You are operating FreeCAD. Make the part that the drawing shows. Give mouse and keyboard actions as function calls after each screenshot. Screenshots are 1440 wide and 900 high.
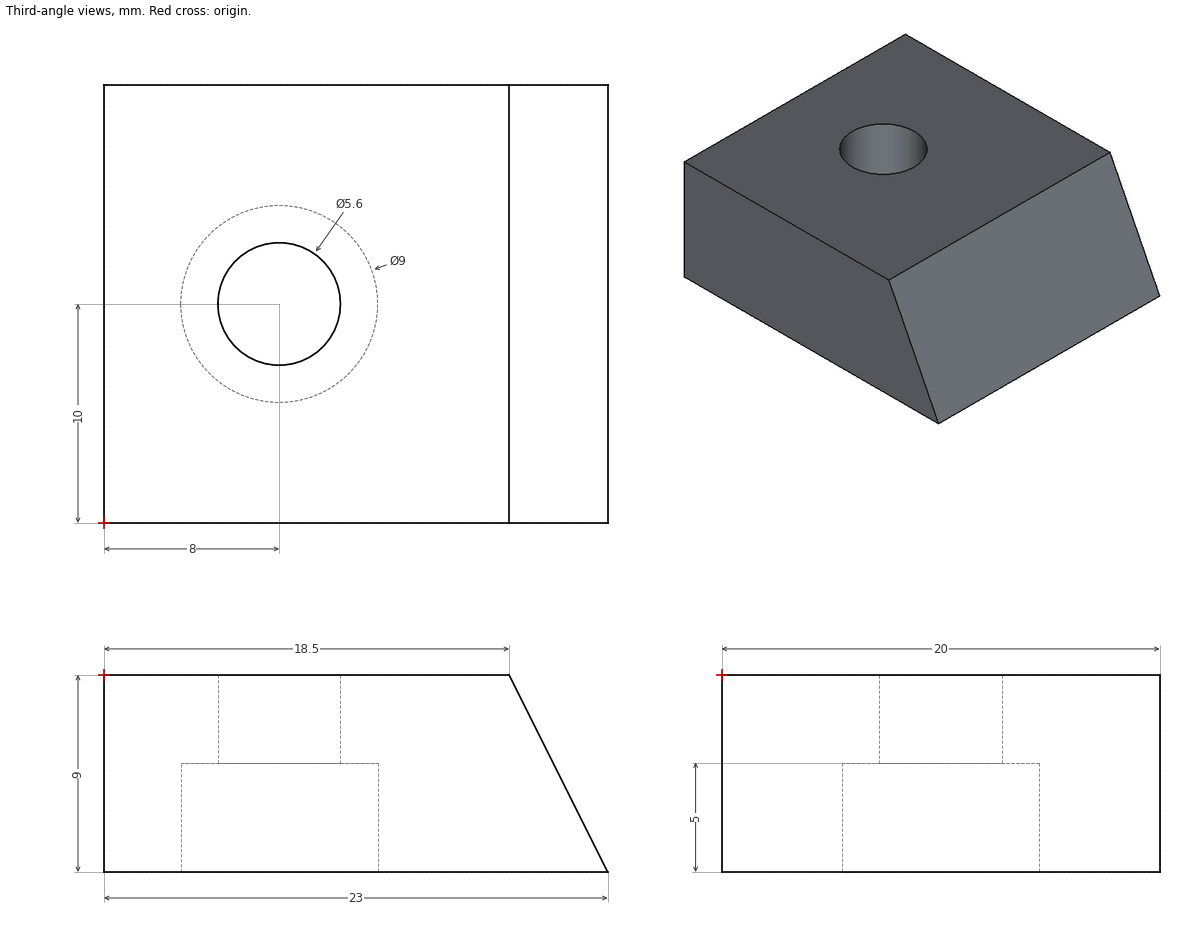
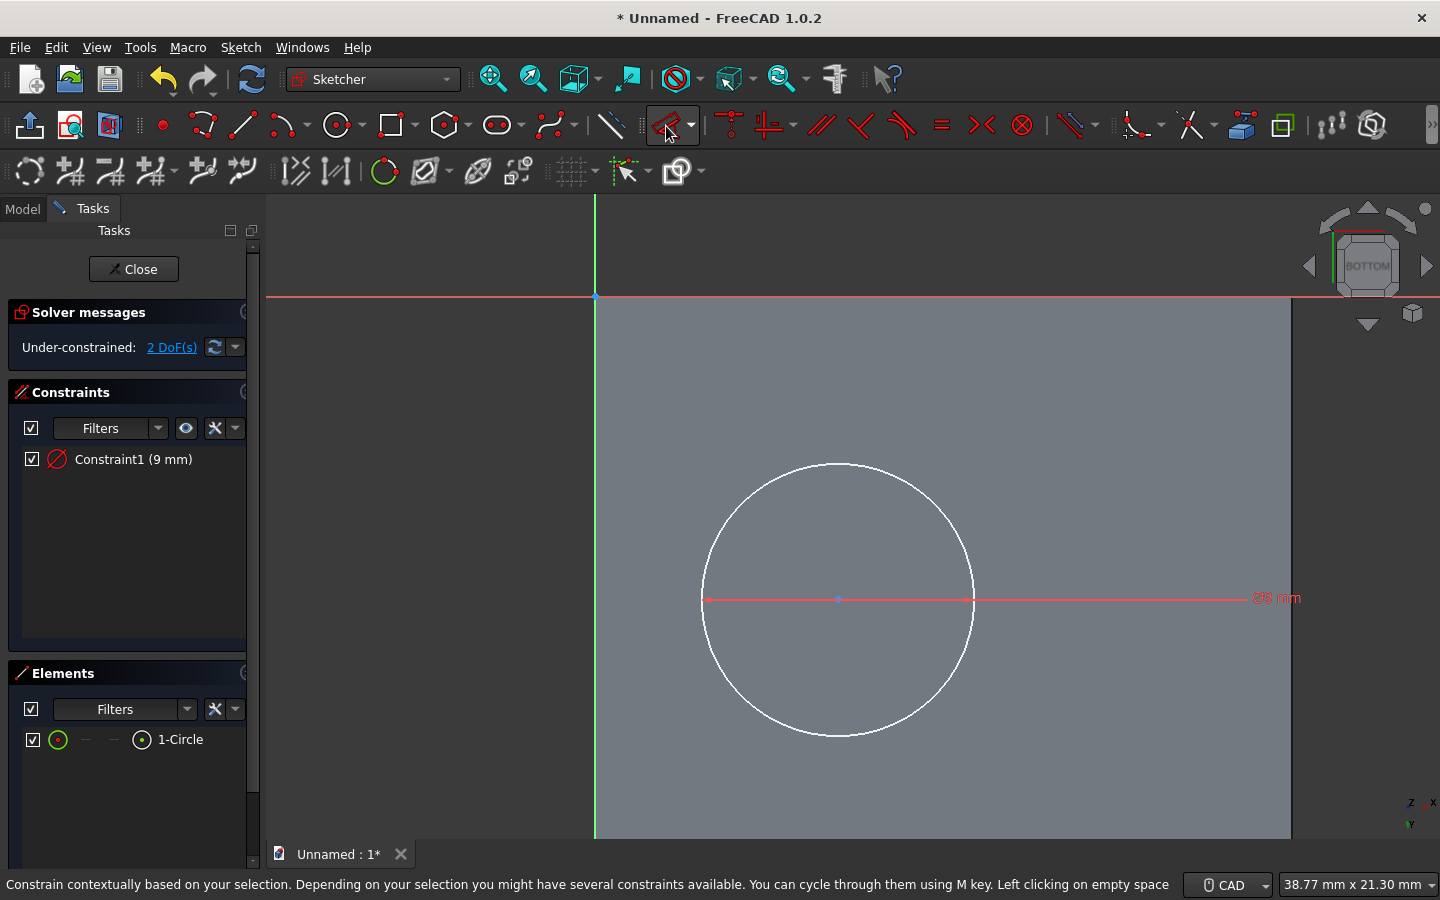
click(838, 600)
click(717, 263)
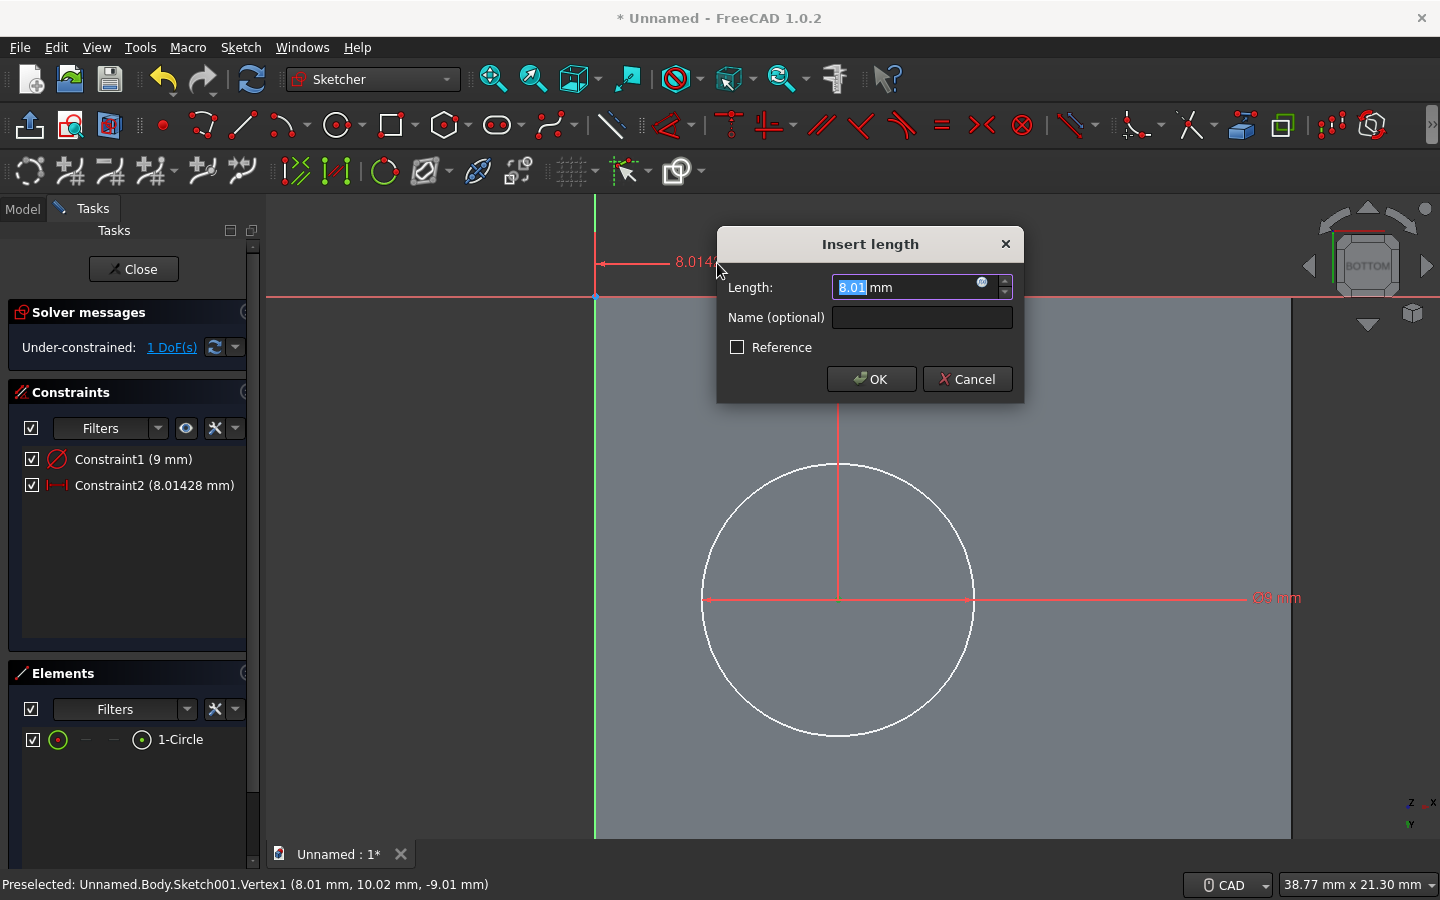
text(8)
key(Return)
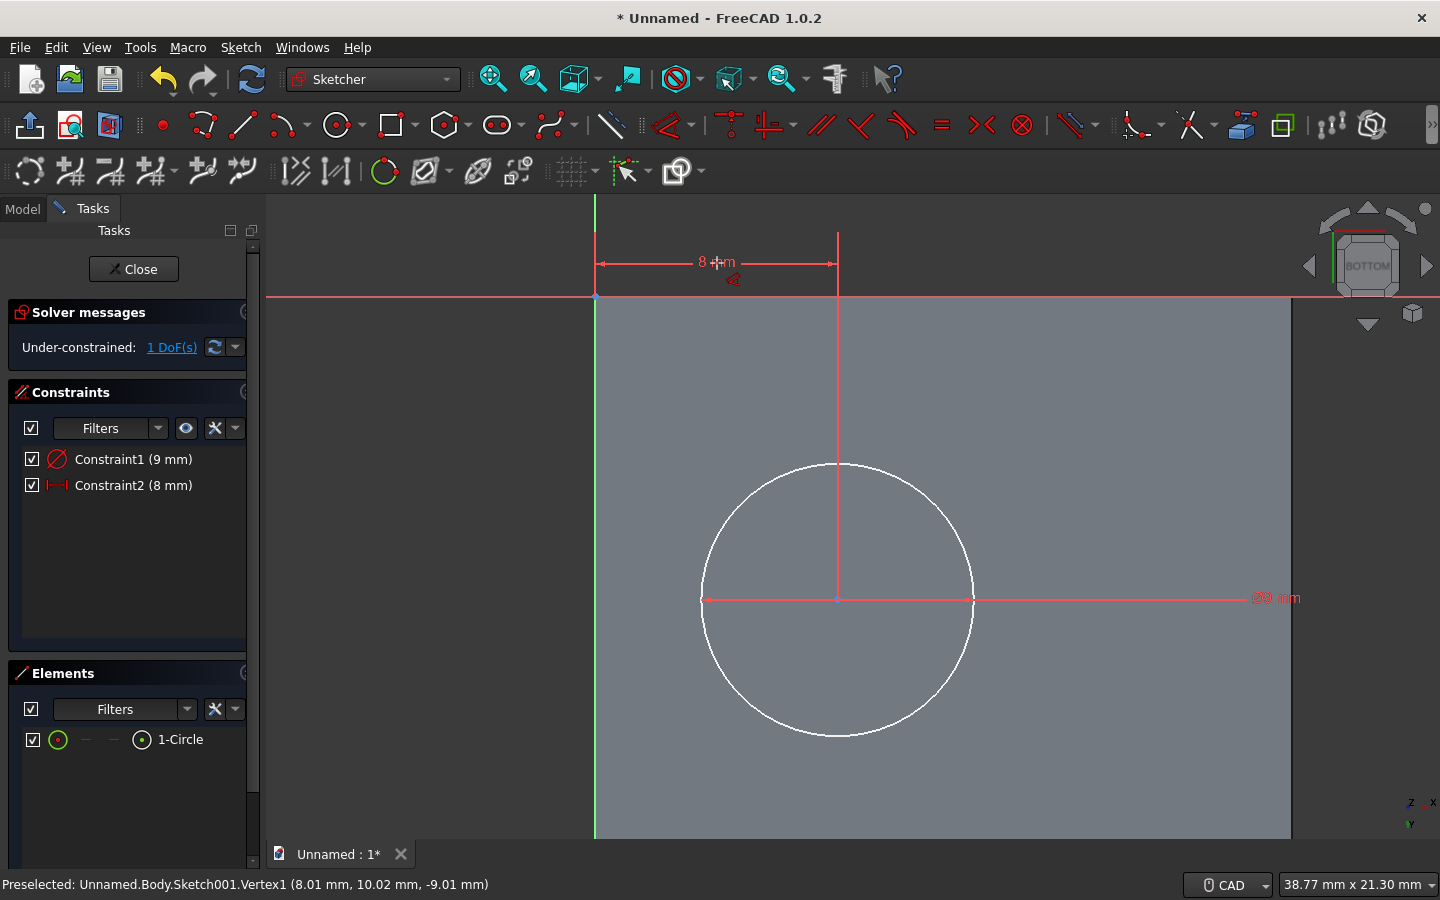
click(838, 600)
click(561, 448)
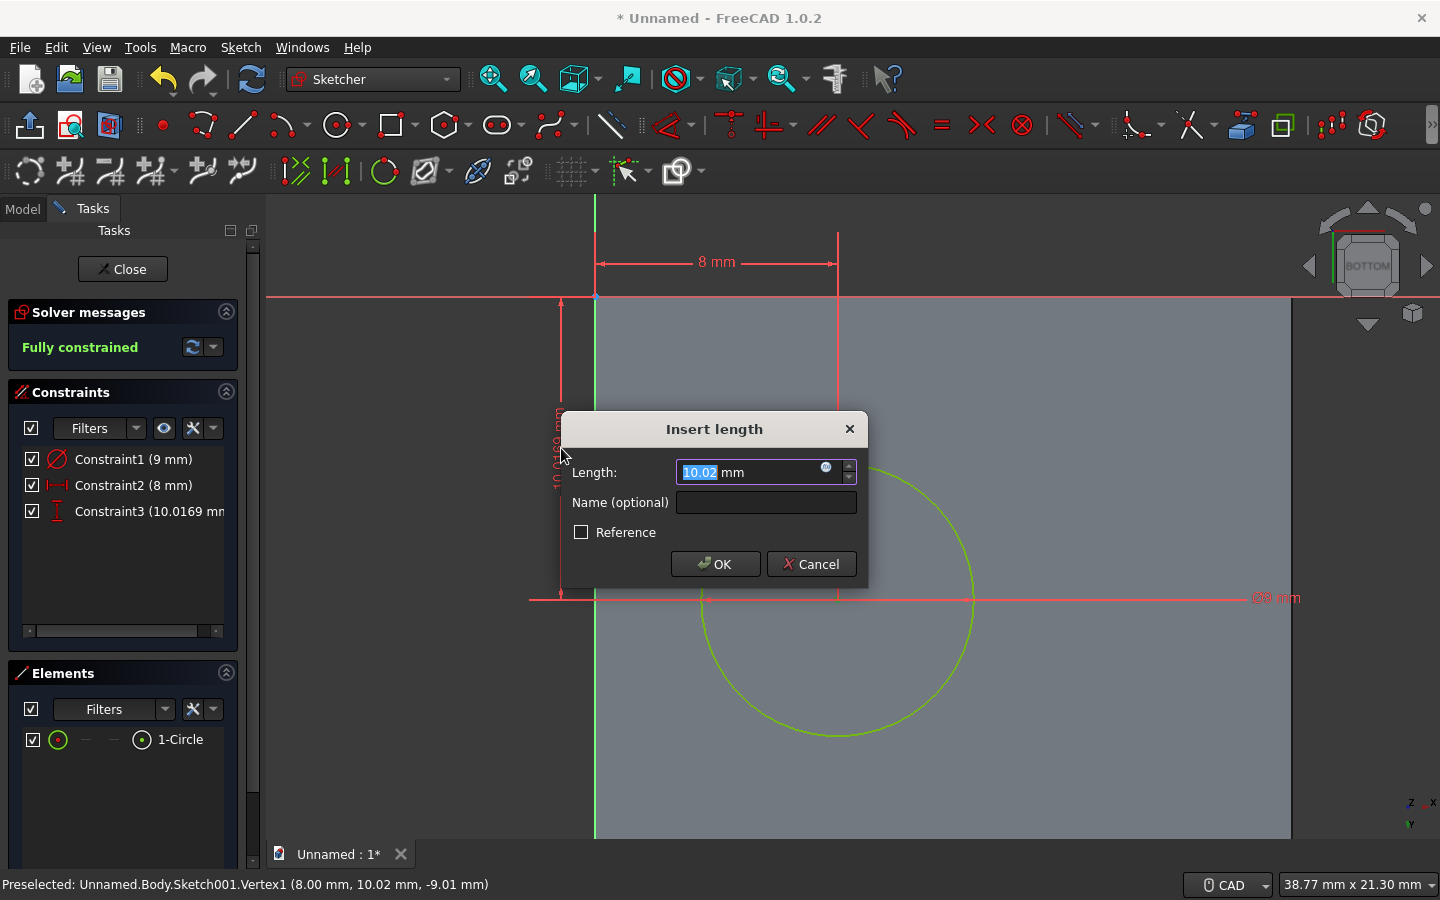
text(10)
key(Return)
key(Escape)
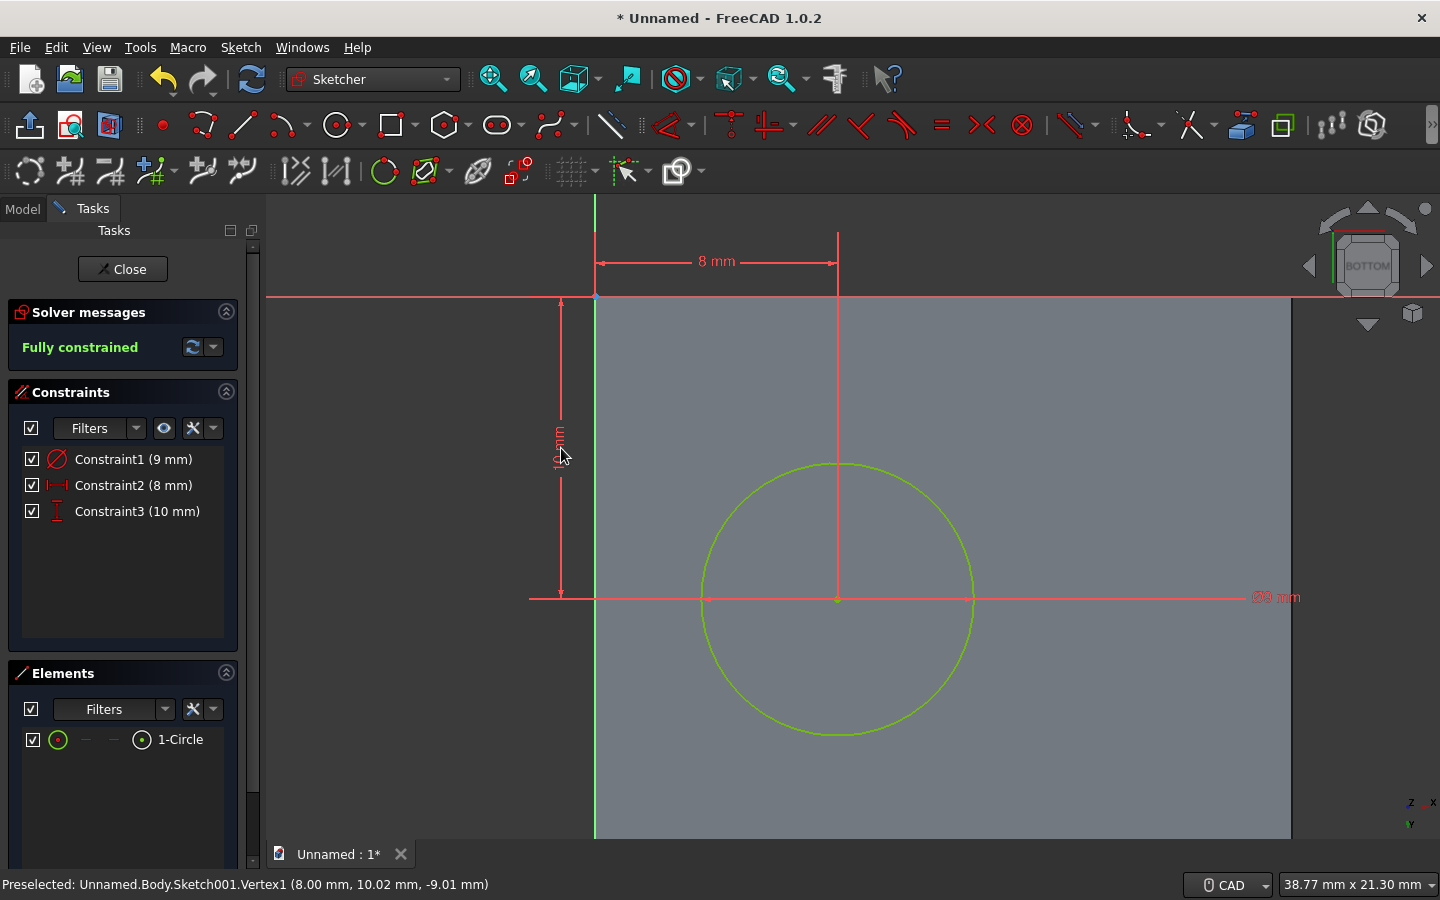
click(123, 269)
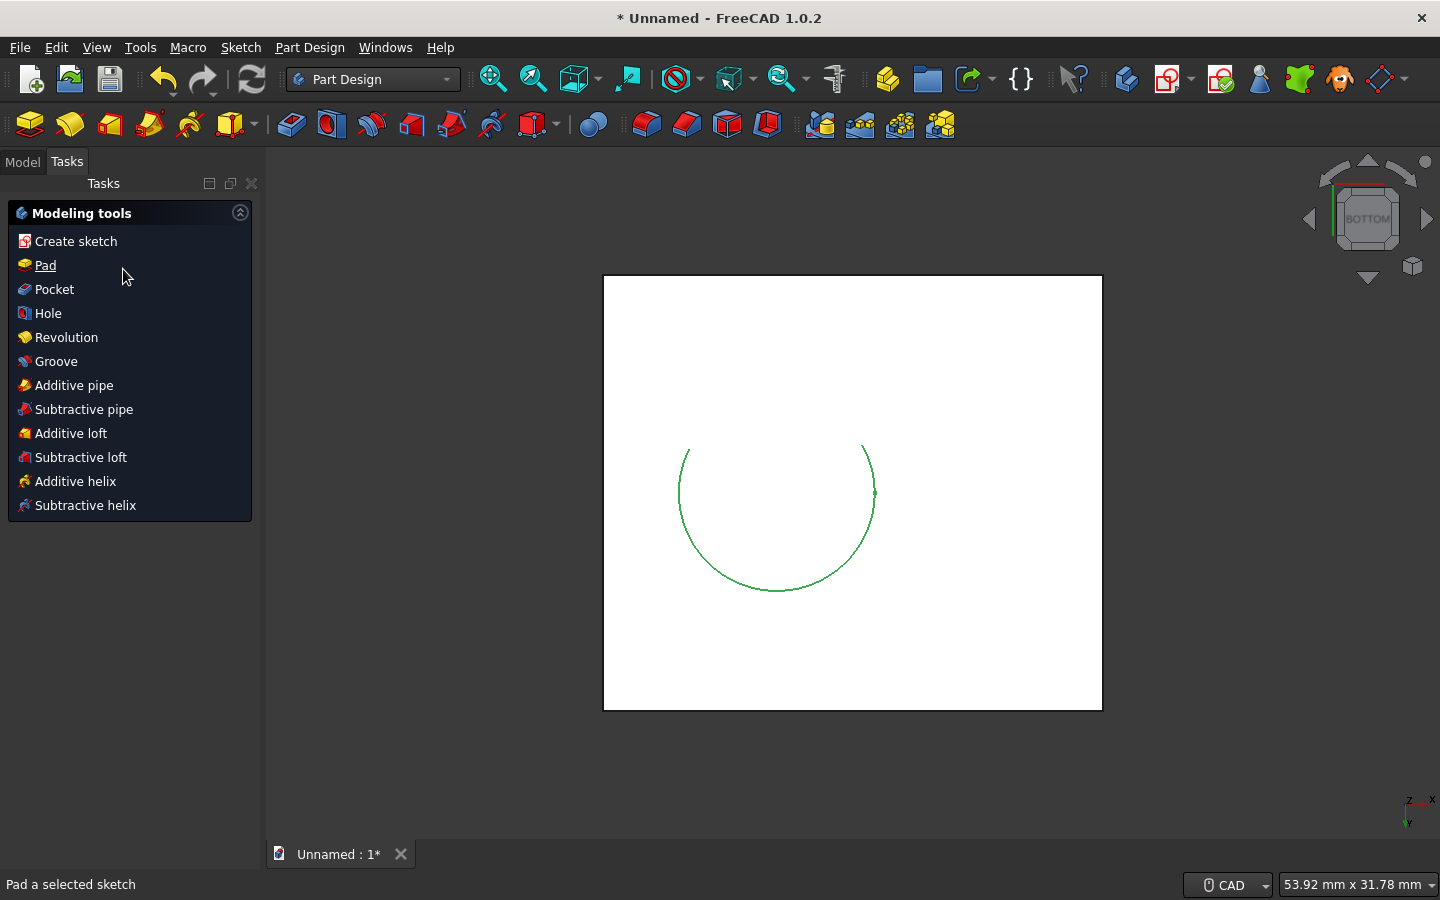
click(292, 124)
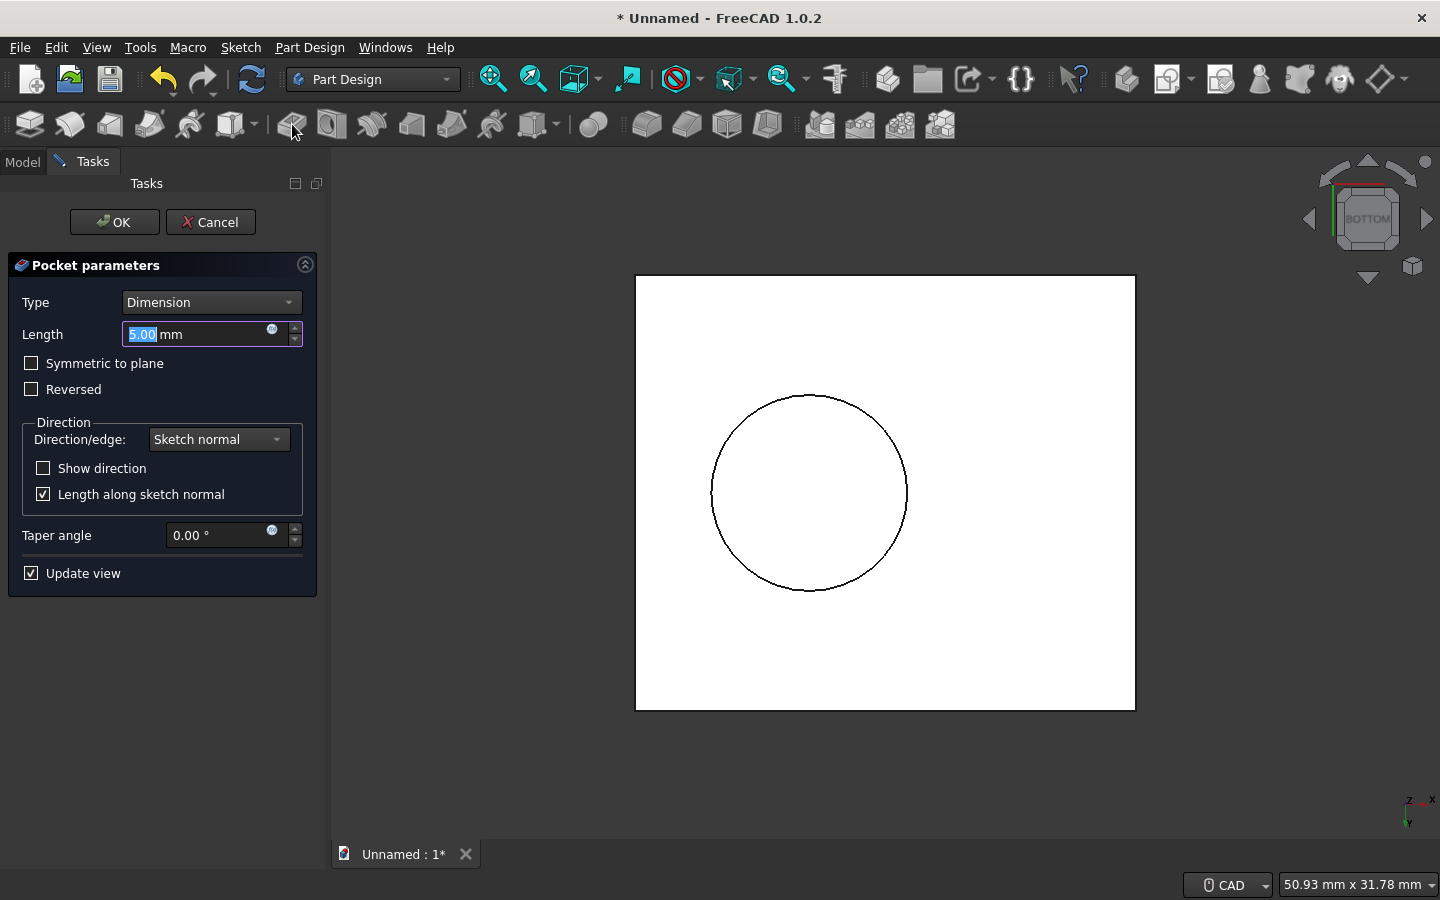
text(5)
key(Tab)